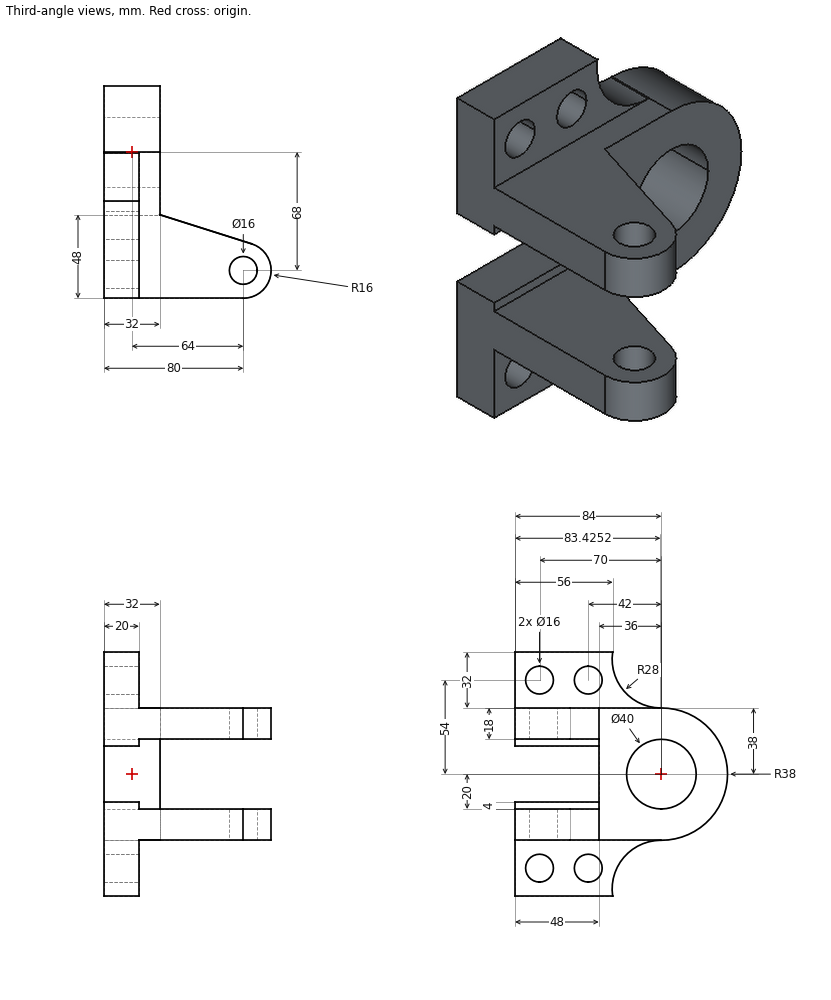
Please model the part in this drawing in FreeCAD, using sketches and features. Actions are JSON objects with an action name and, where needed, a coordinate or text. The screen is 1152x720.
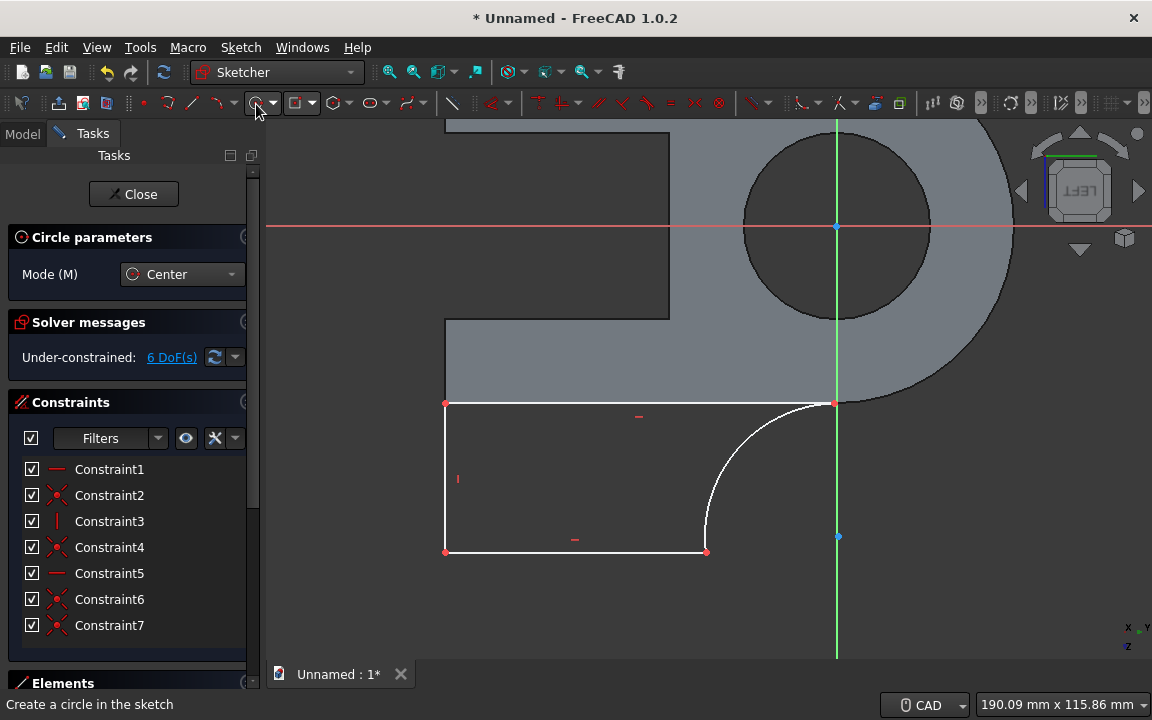
{"action": "left_click", "coordinate": [511, 478]}
{"action": "left_click", "coordinate": [537, 451]}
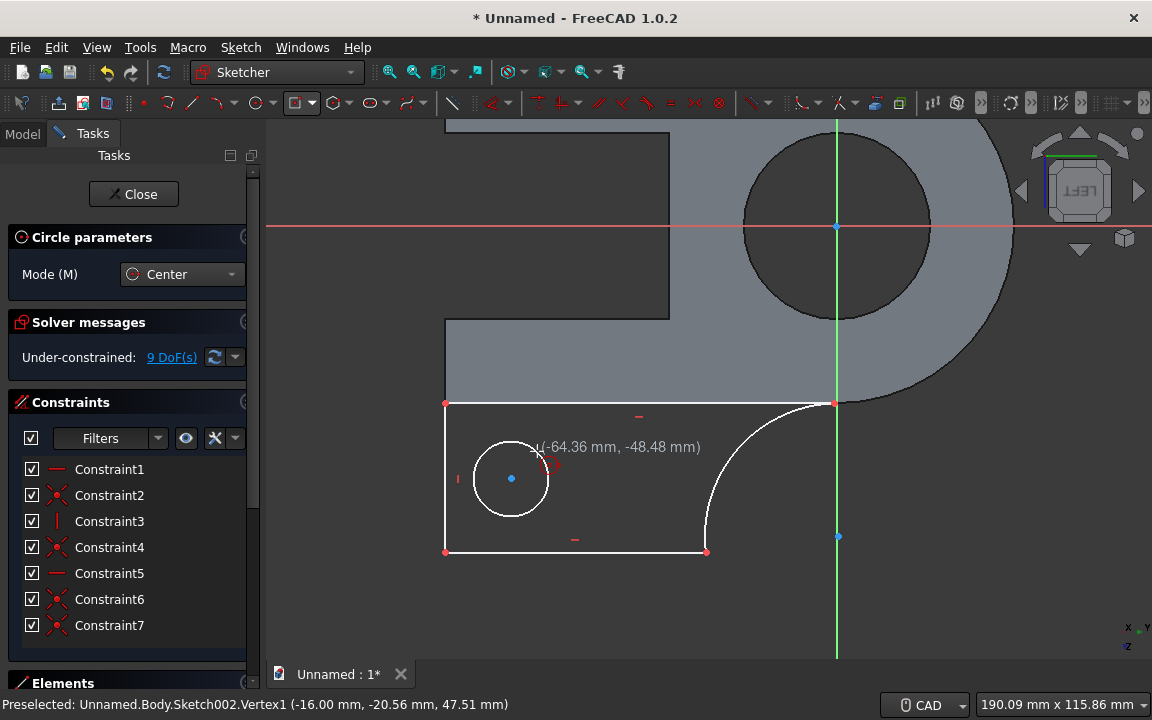
{"action": "left_click", "coordinate": [641, 478]}
{"action": "left_click", "coordinate": [668, 451]}
{"action": "key", "text": "Escape"}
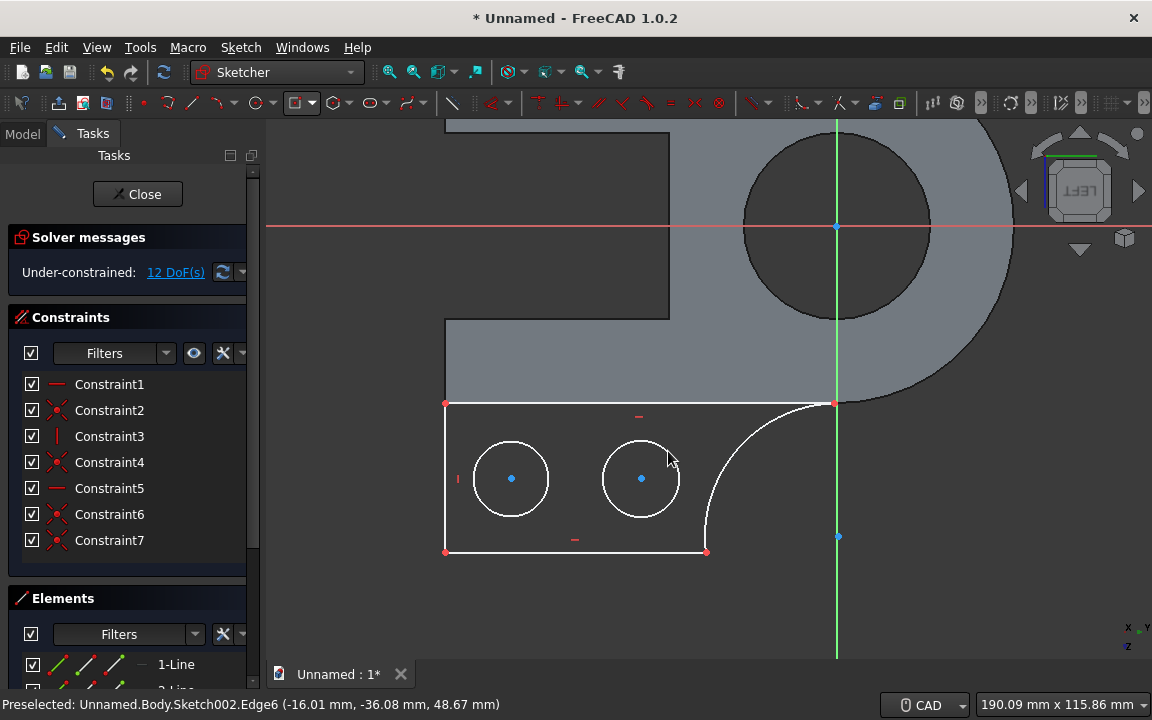
{"action": "left_click", "coordinate": [537, 452]}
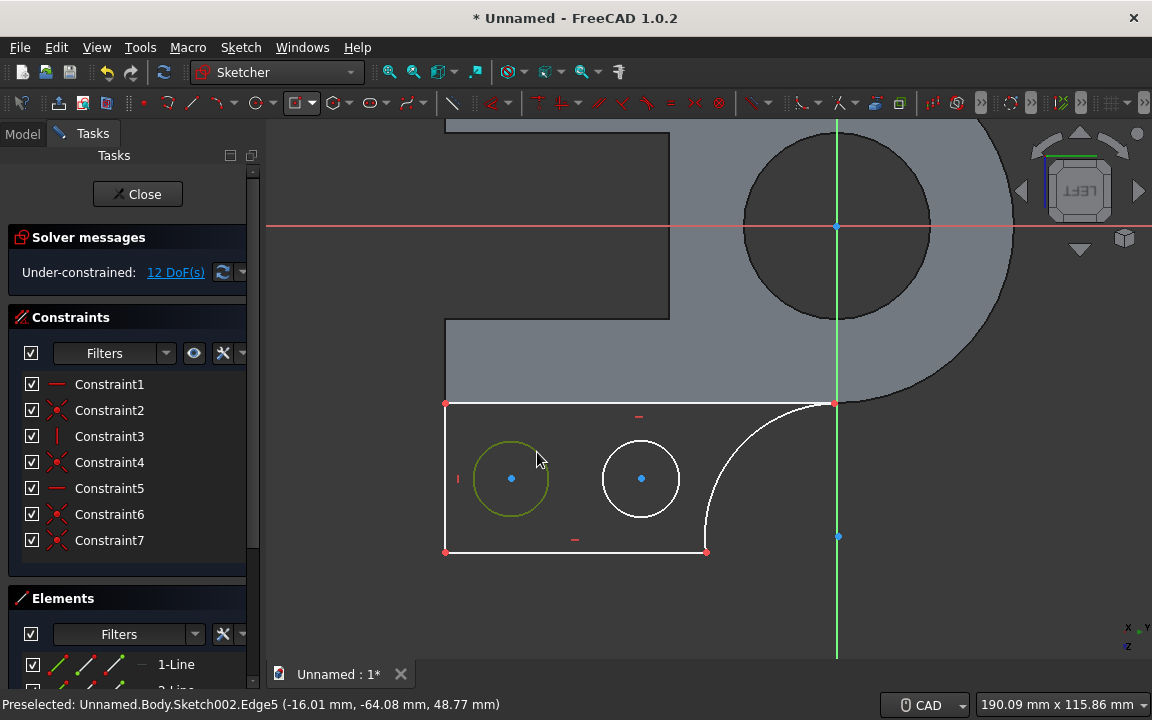
{"action": "left_click", "coordinate": [668, 452]}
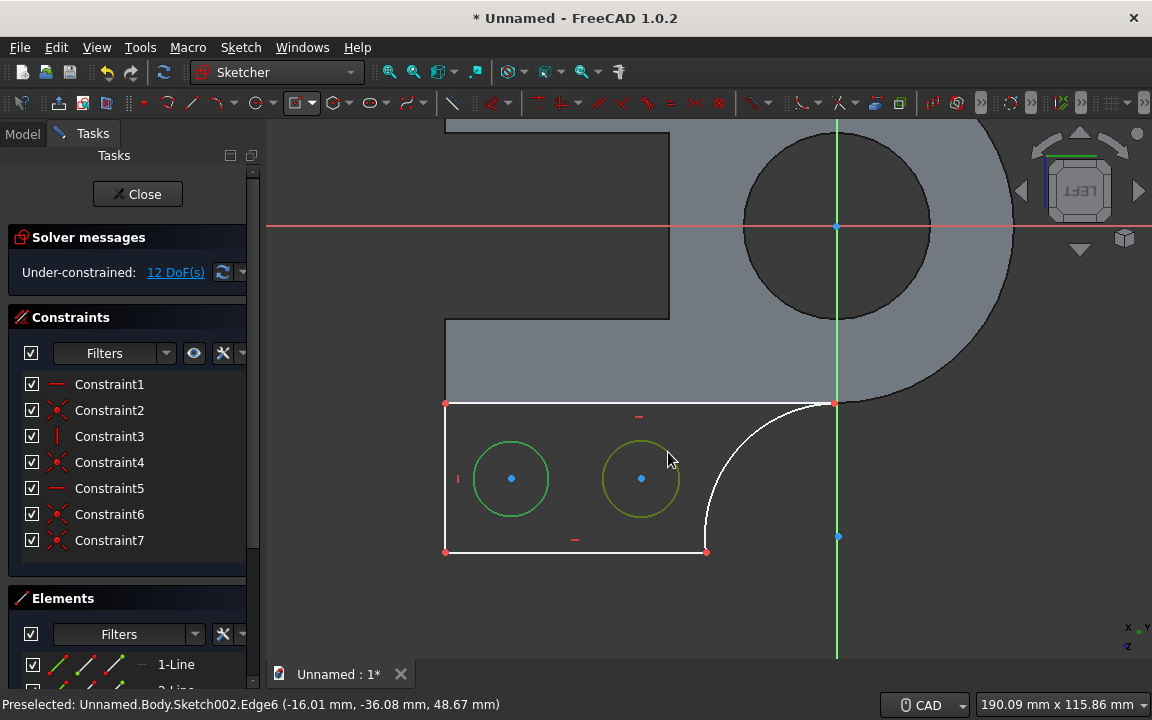
{"action": "key", "text": "e"}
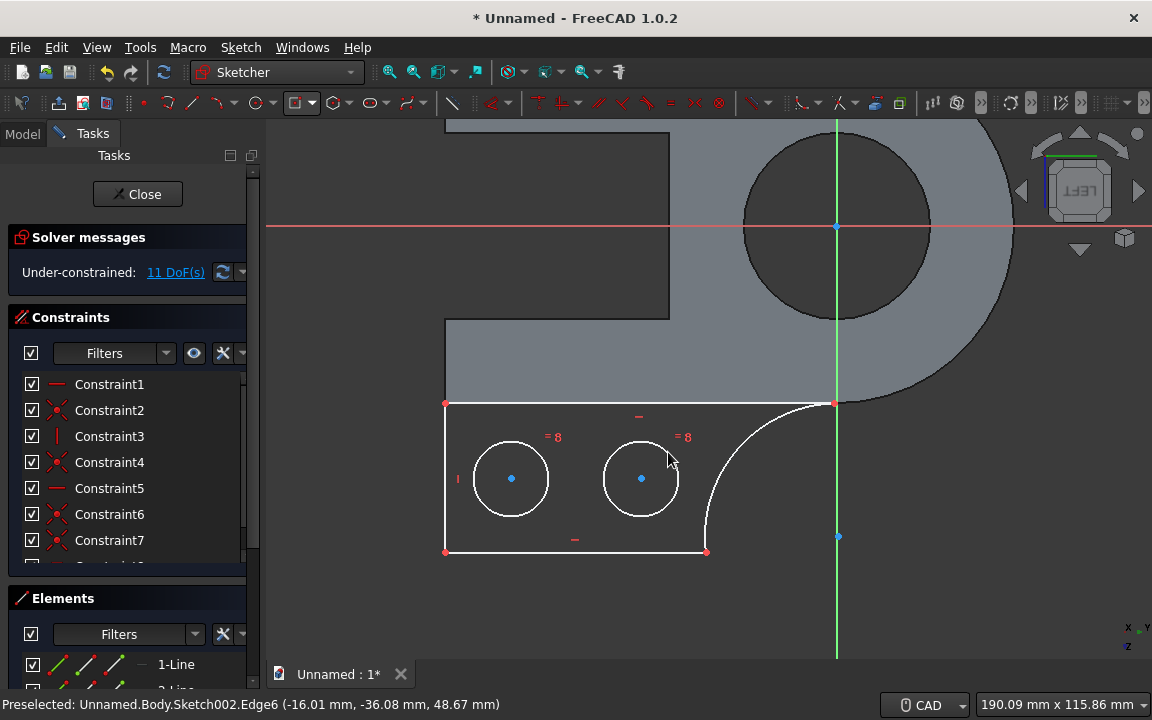
{"action": "left_click", "coordinate": [511, 479]}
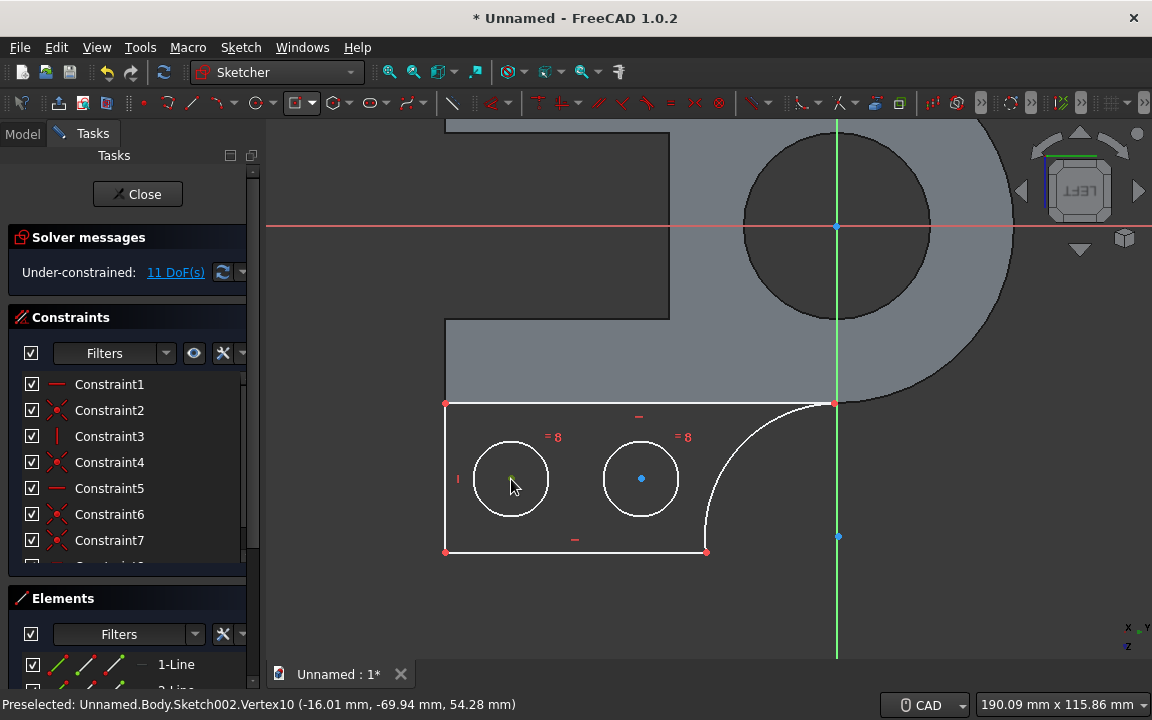
{"action": "left_click", "coordinate": [641, 479]}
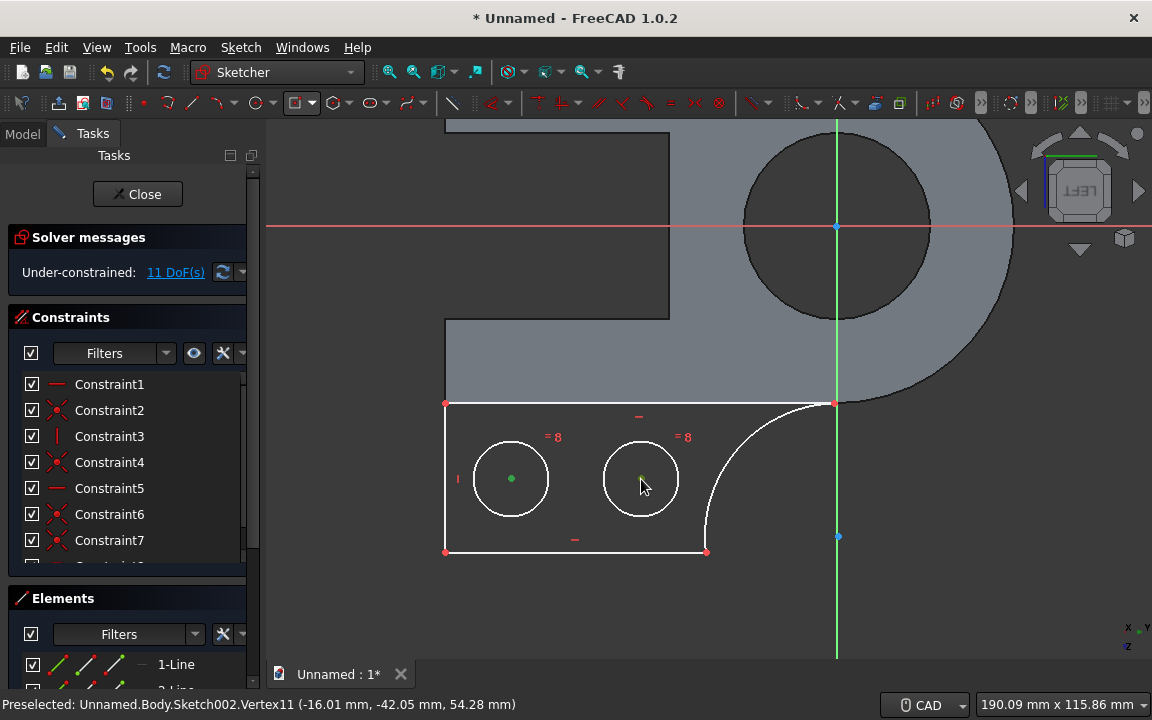
{"action": "key", "text": "h"}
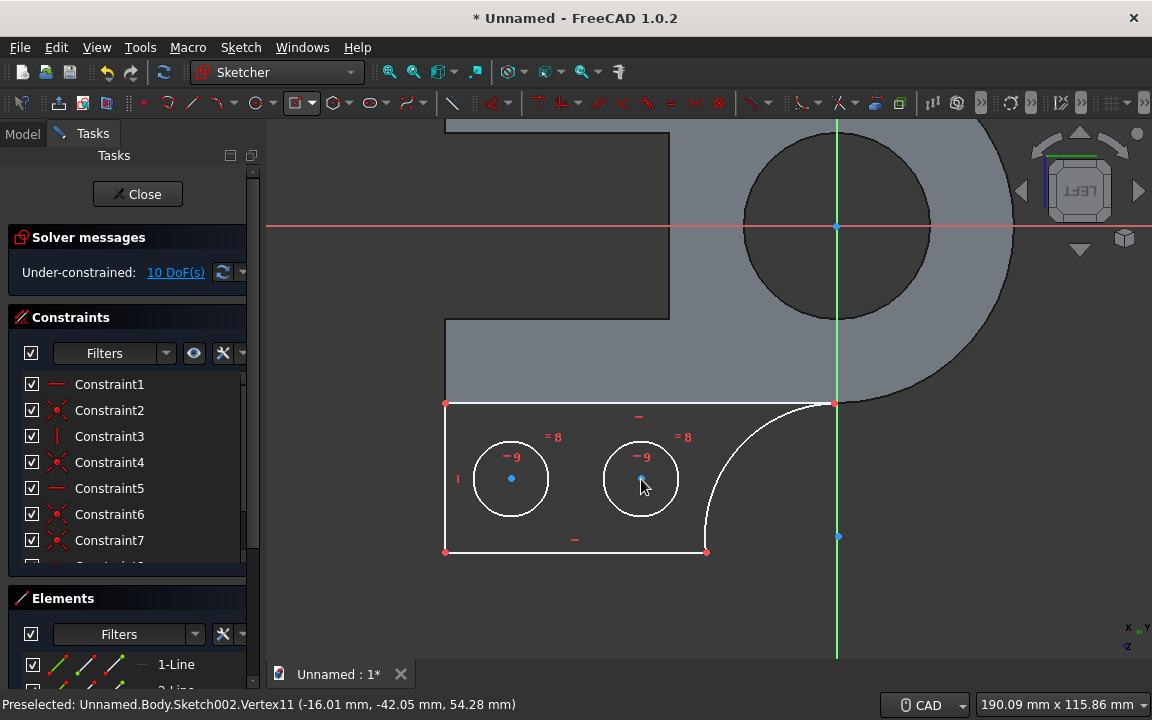
{"action": "left_click", "coordinate": [492, 104]}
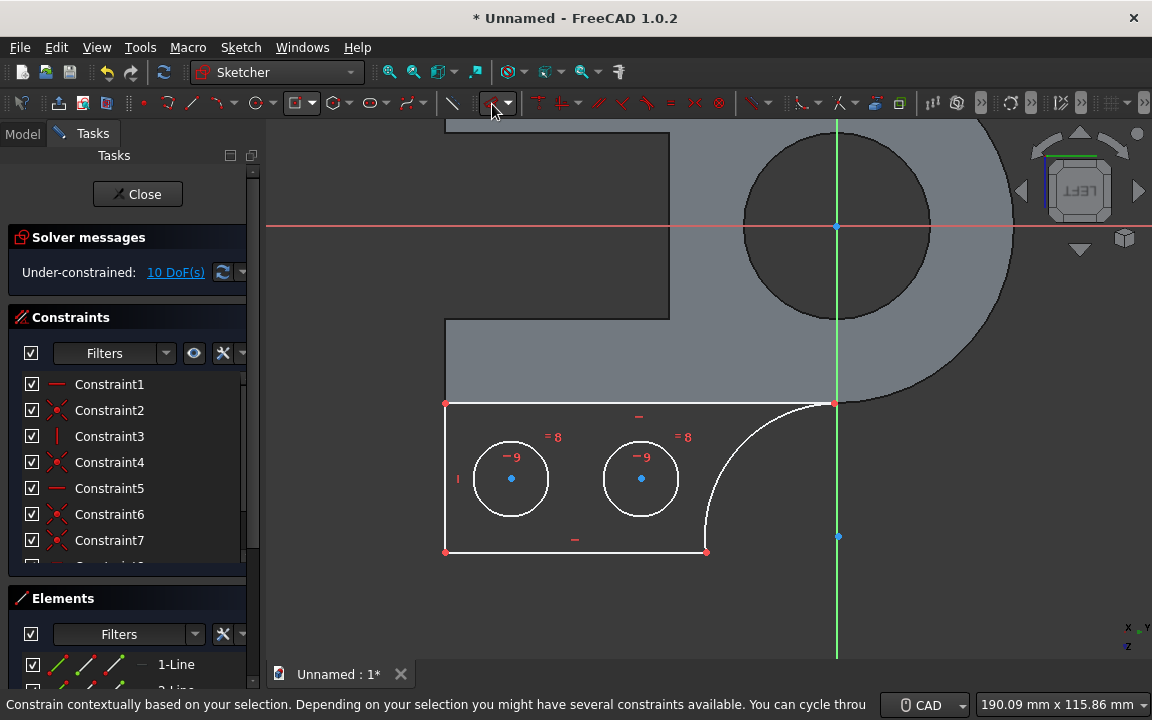
{"action": "left_click", "coordinate": [771, 422]}
{"action": "left_click", "coordinate": [697, 452]}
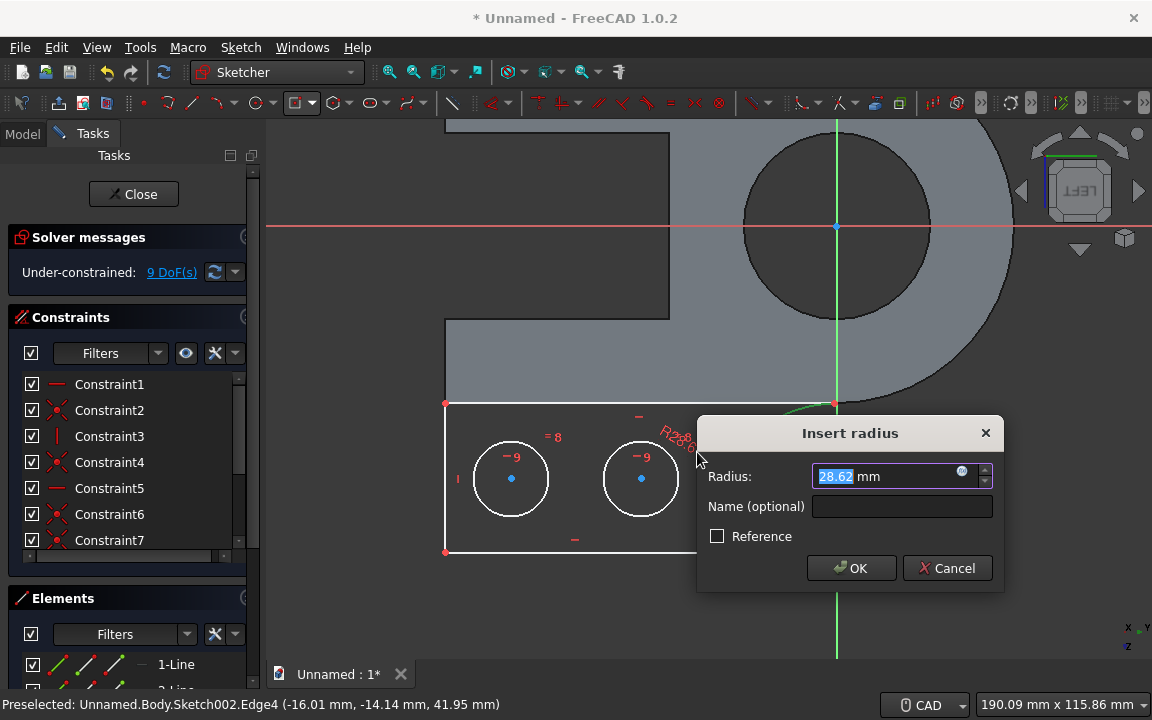
{"action": "type", "text": "28"}
{"action": "key", "text": "Return"}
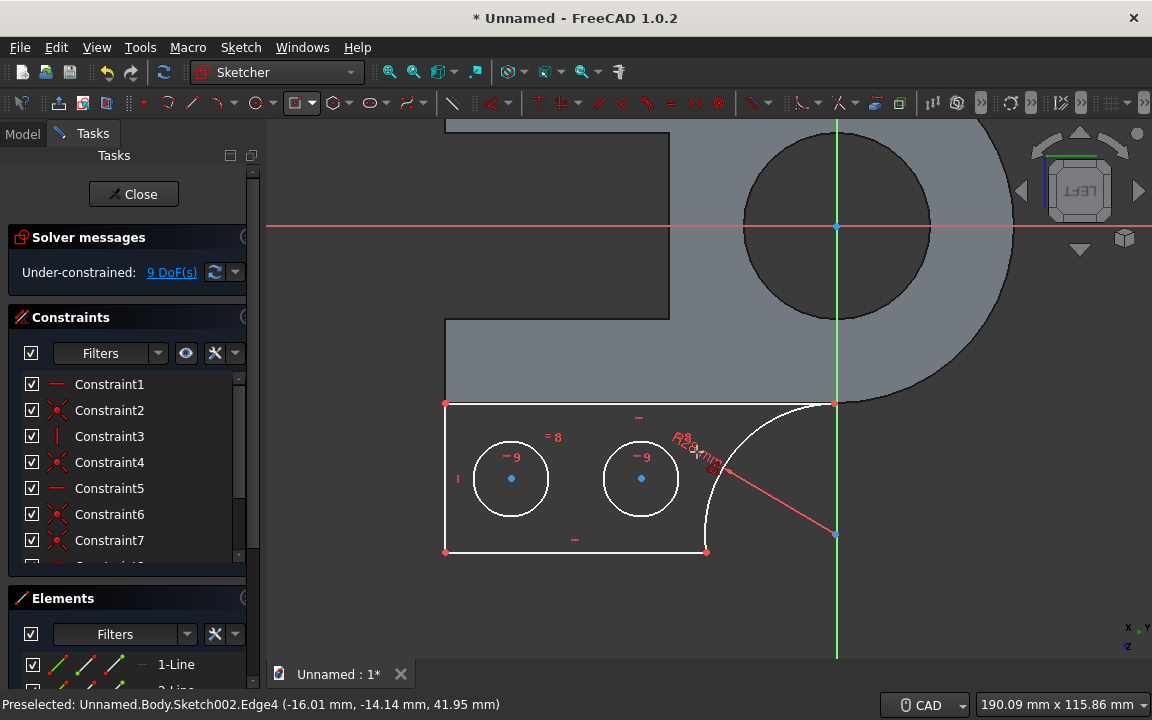
{"action": "left_click", "coordinate": [537, 452]}
{"action": "left_click", "coordinate": [559, 429]}